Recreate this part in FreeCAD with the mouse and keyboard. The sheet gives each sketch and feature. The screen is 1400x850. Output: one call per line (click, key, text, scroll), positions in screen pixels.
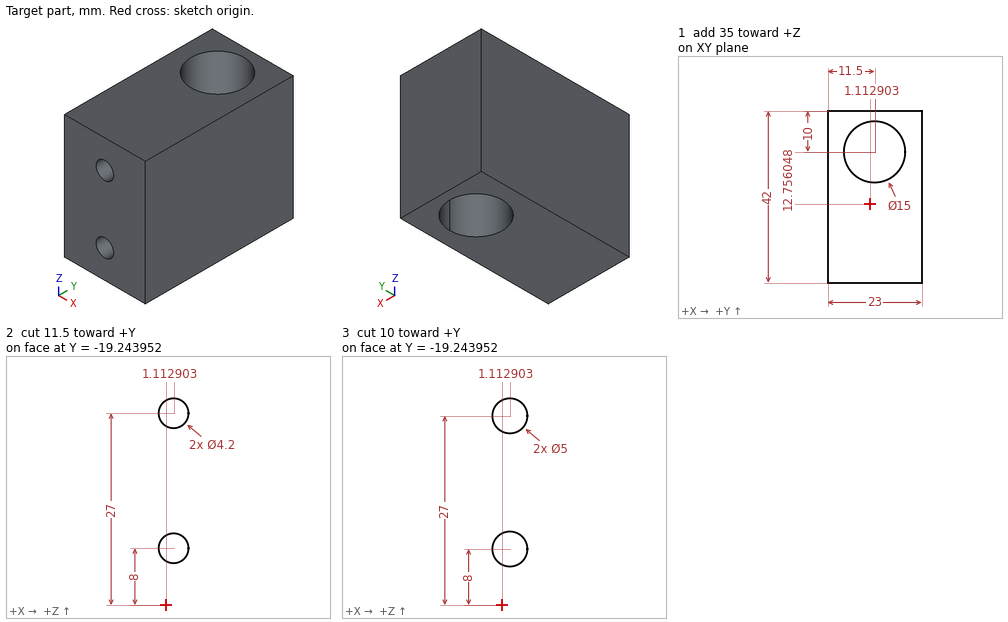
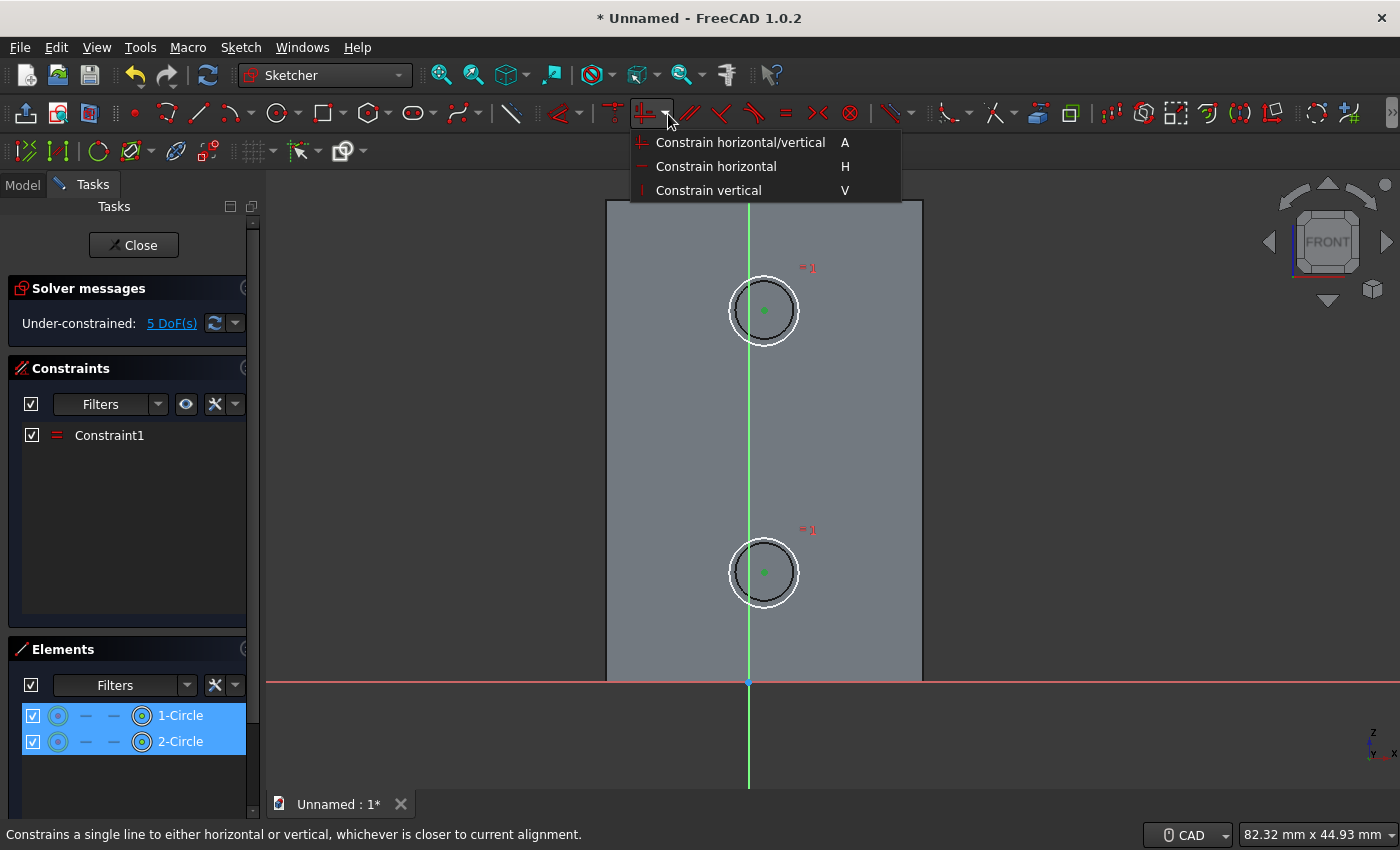
click(766, 190)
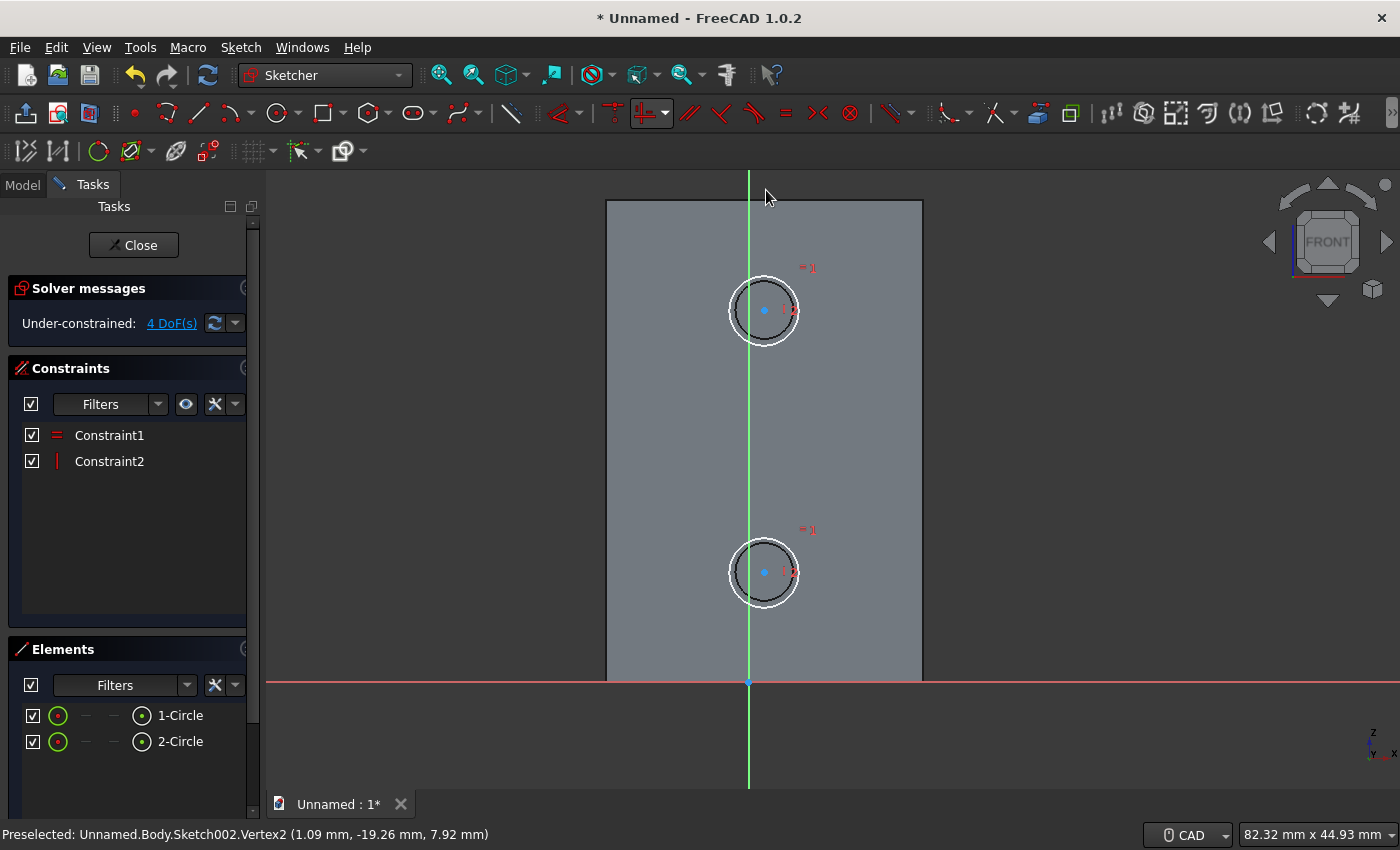
click(558, 114)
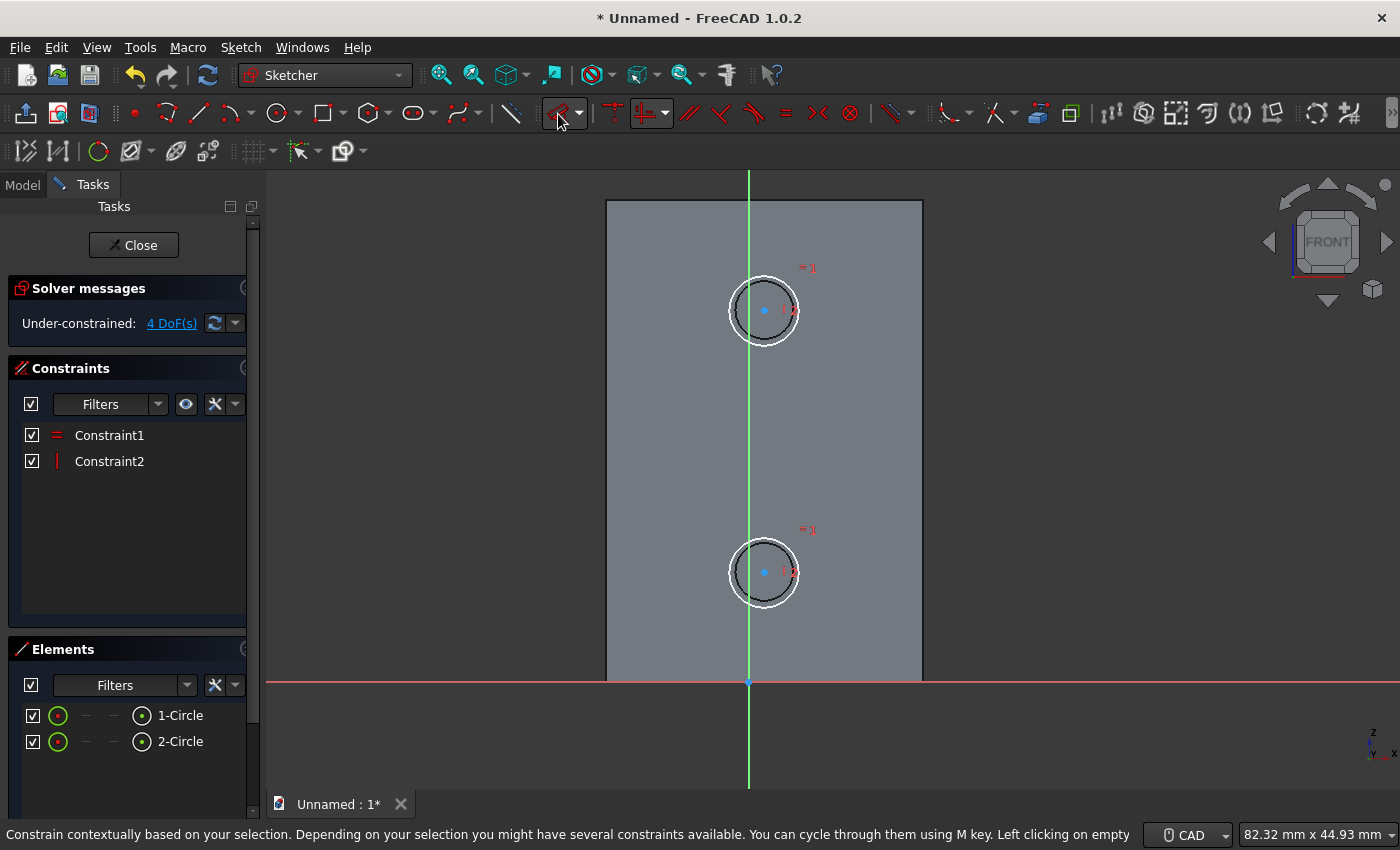
click(788, 286)
click(810, 263)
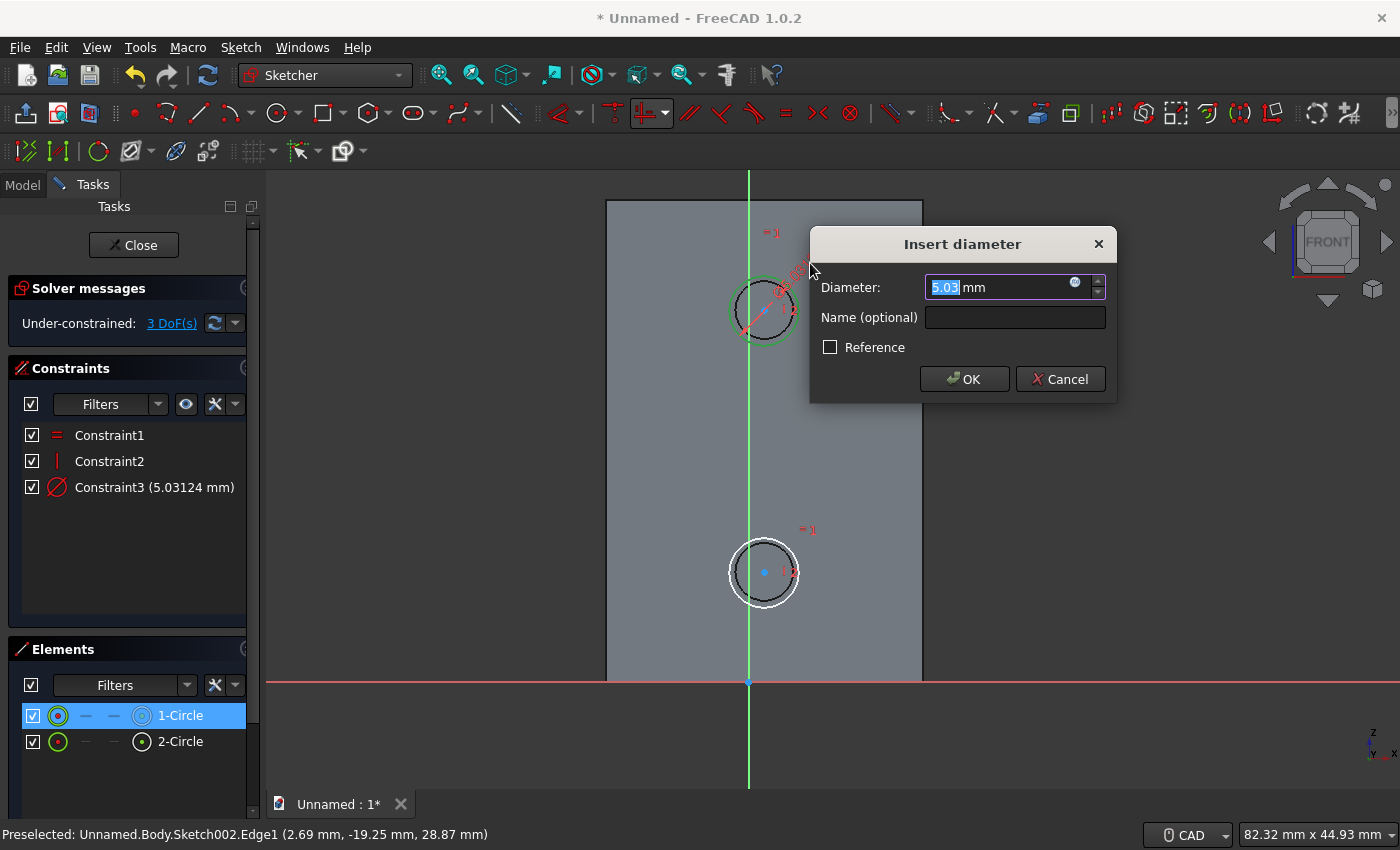
text(5)
key(Return)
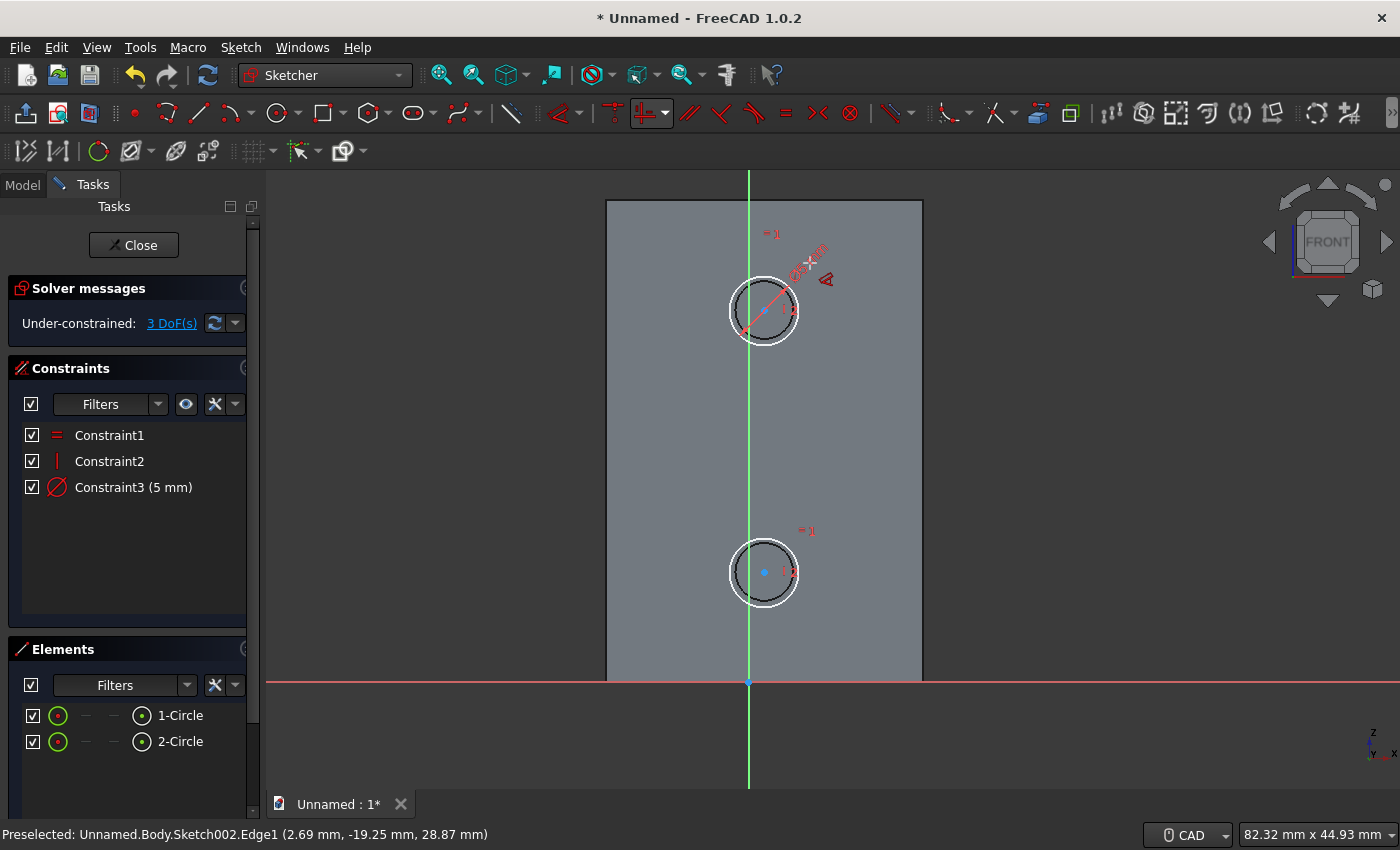
click(764, 573)
click(715, 628)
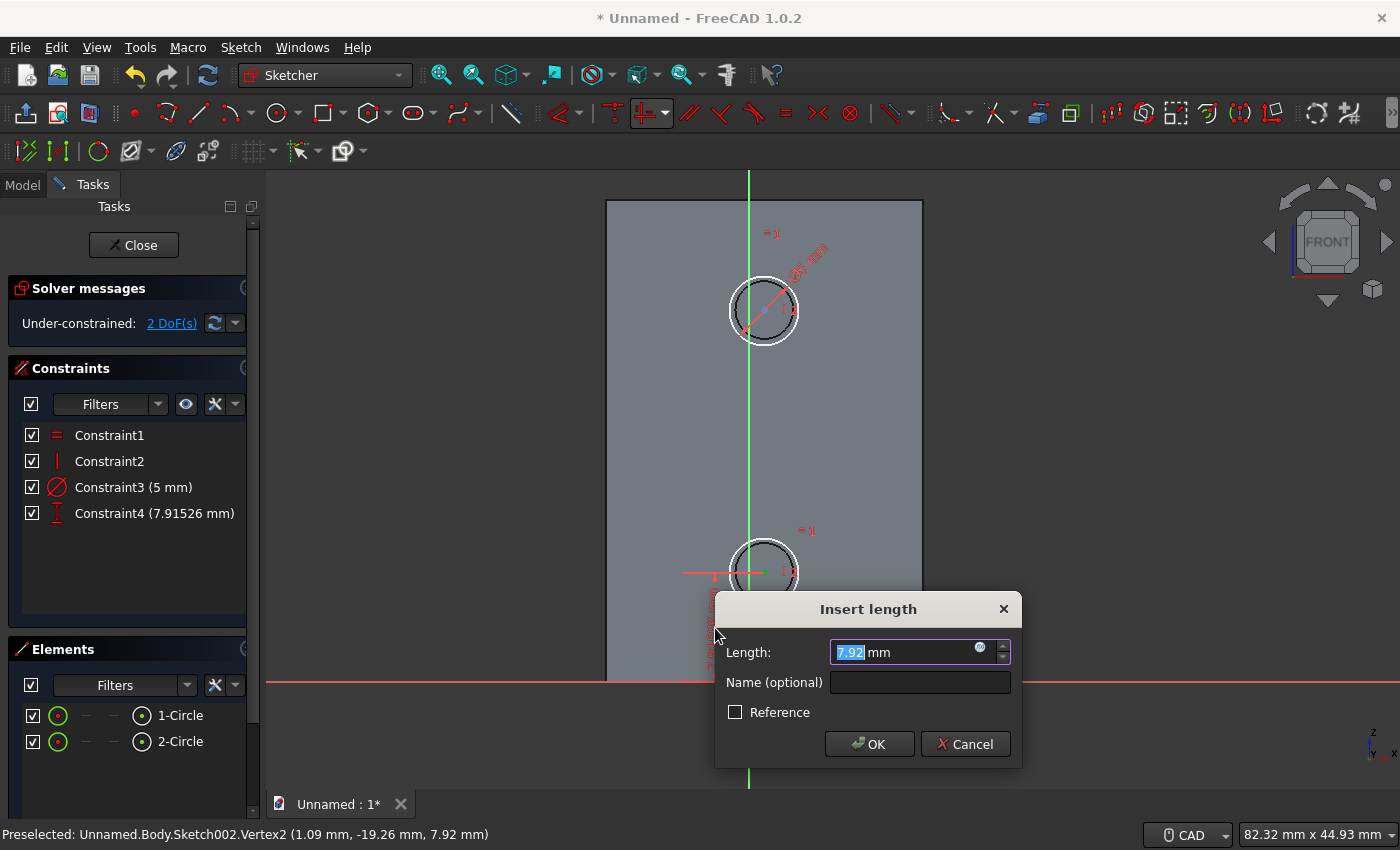
text(8)
key(Return)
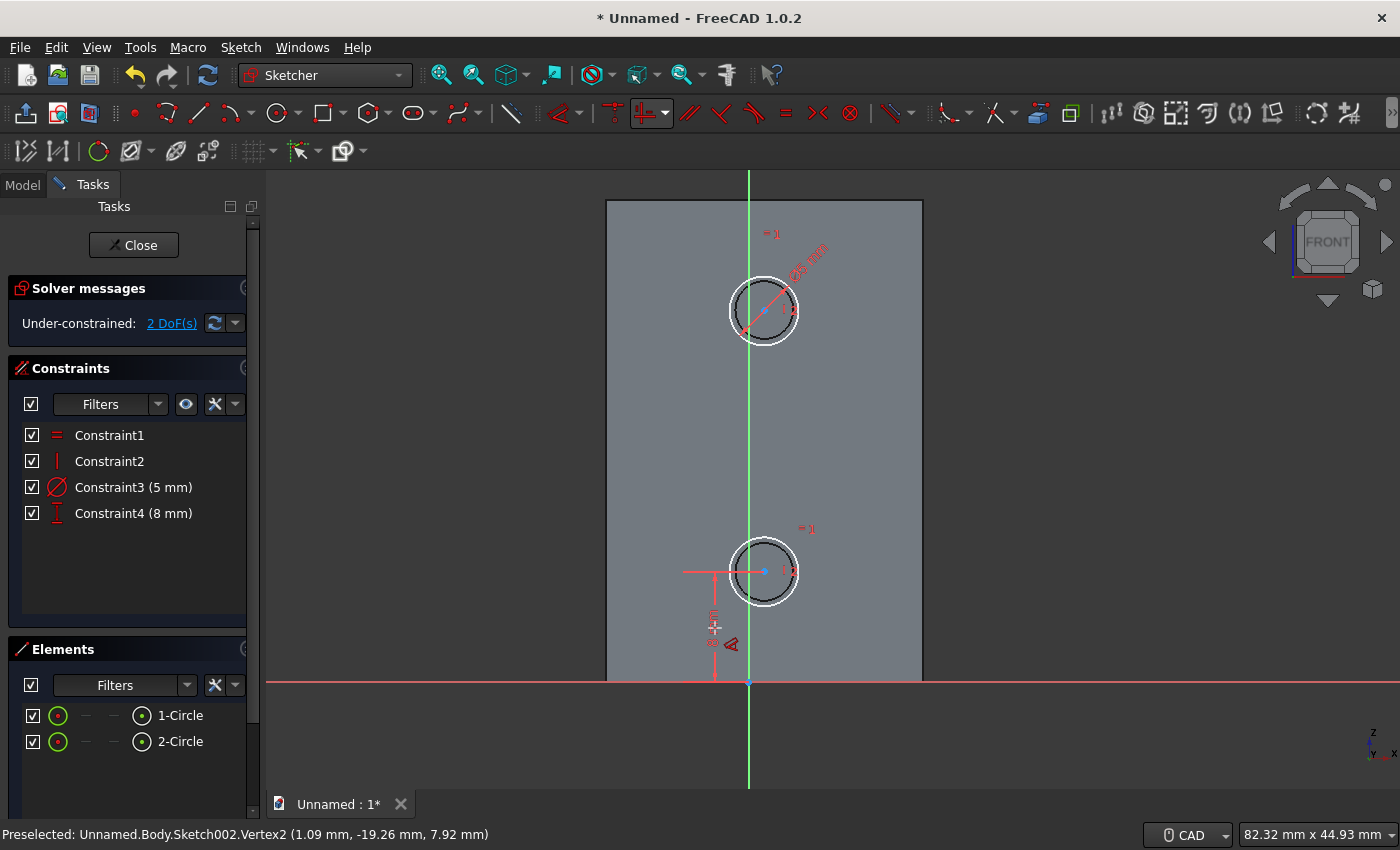
click(764, 311)
click(715, 497)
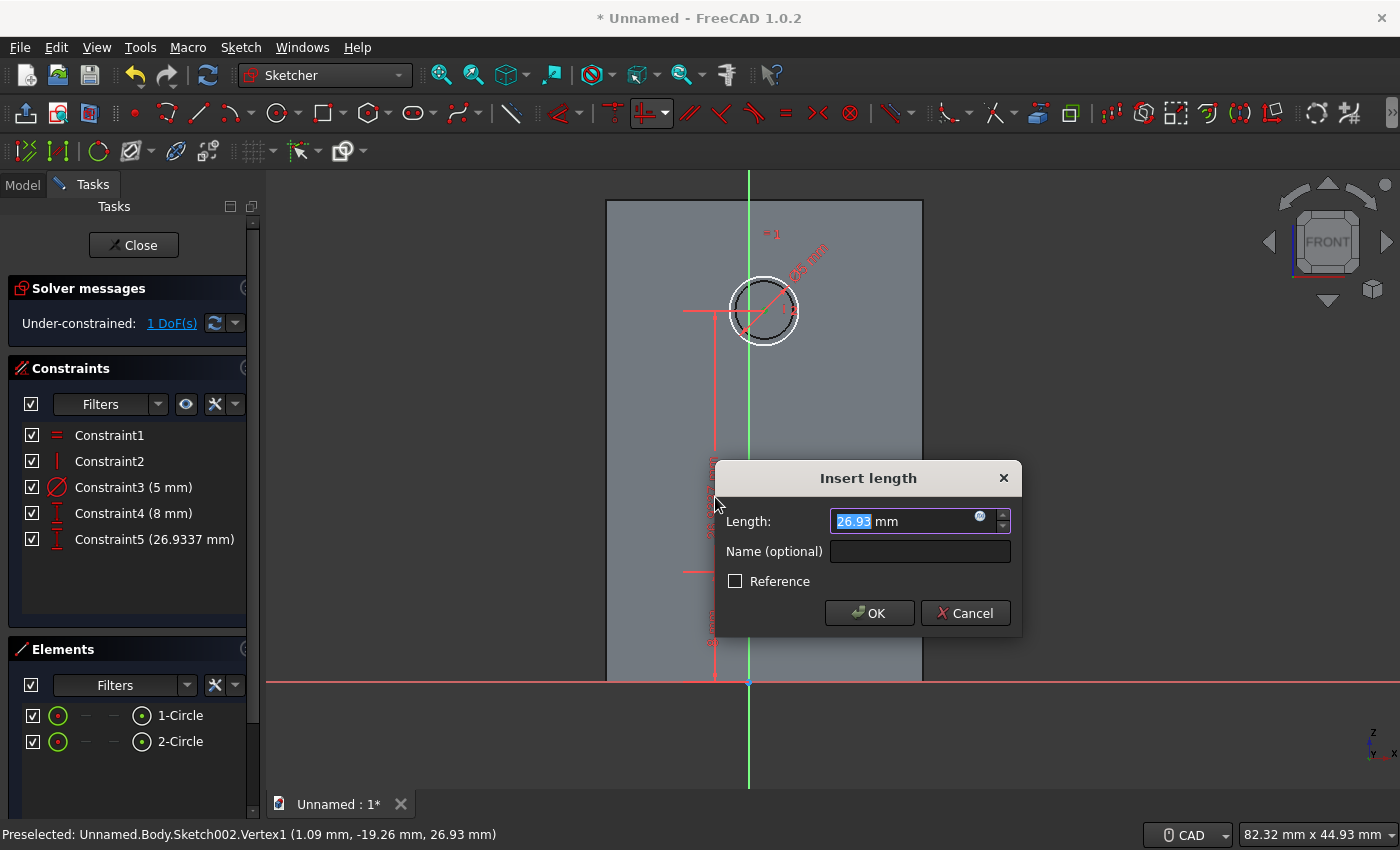
text(27)
key(Return)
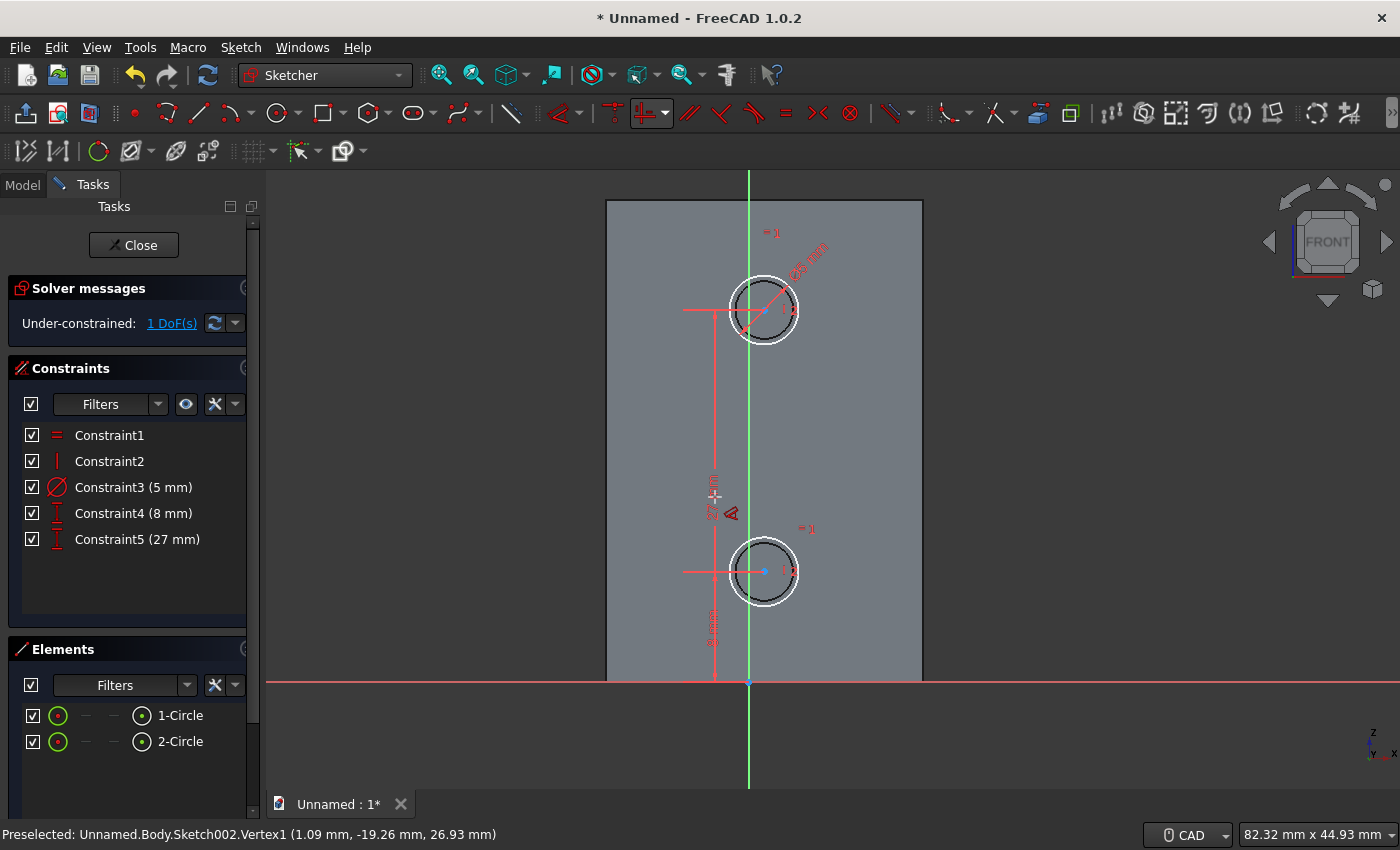
scroll(764, 310, up, 5)